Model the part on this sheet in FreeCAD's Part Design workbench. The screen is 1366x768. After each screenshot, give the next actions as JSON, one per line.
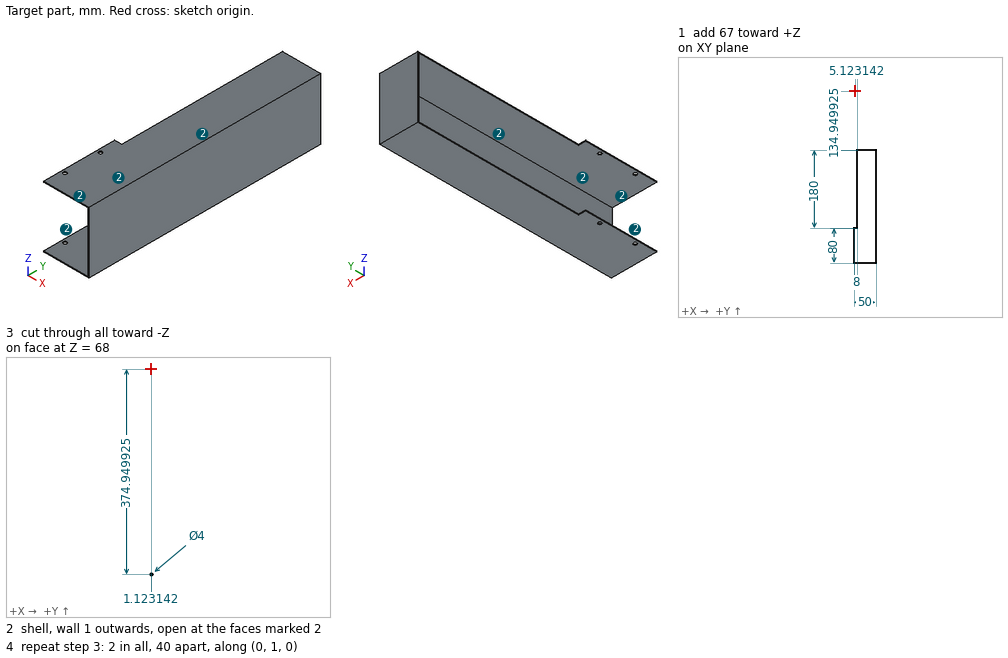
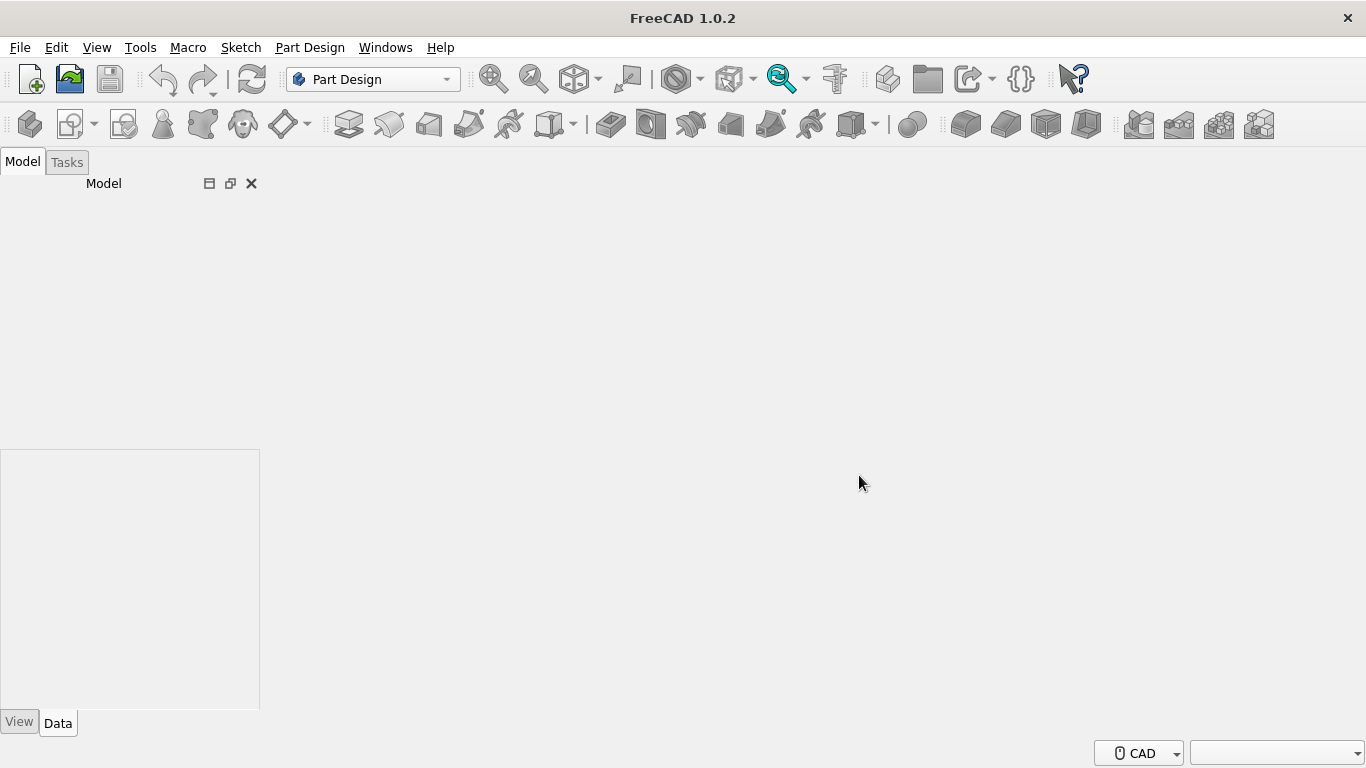
{"action": "left_click", "coordinate": [30, 80]}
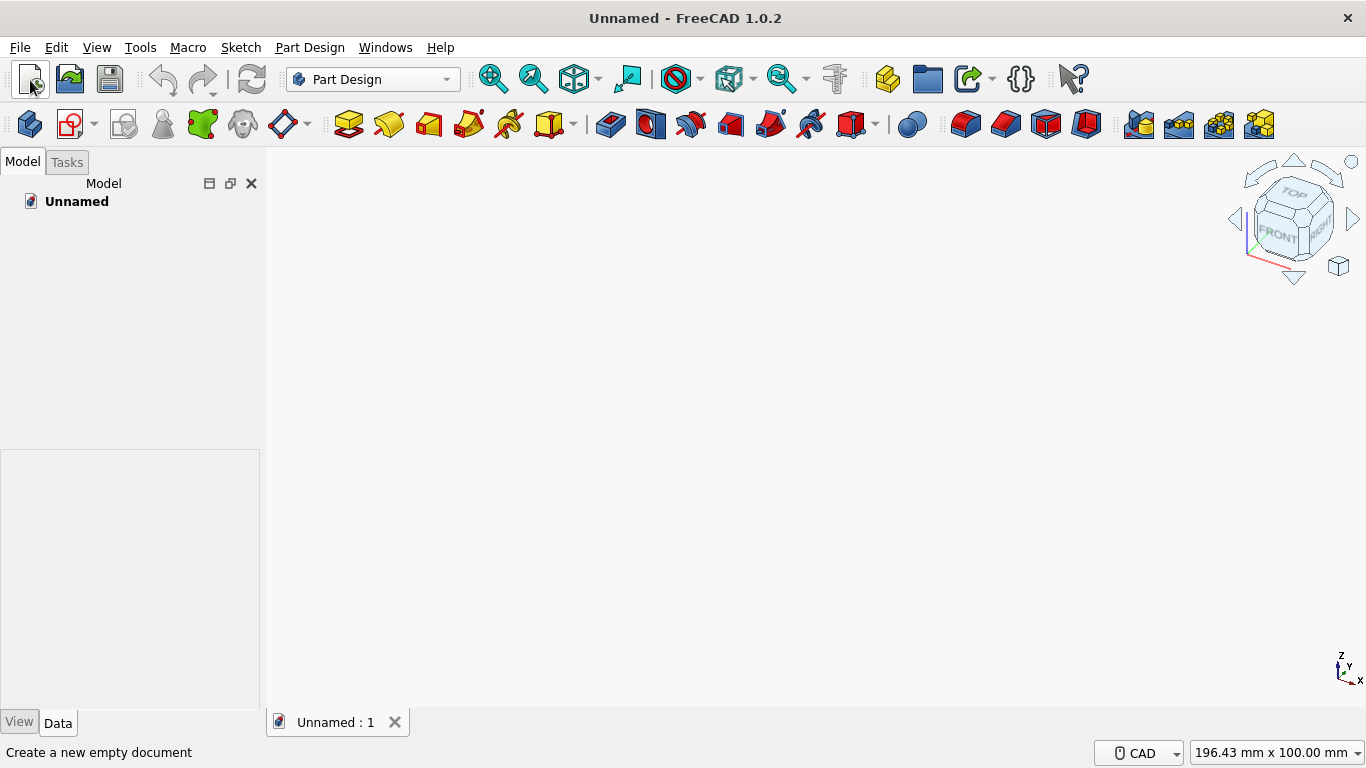
{"action": "left_click", "coordinate": [70, 124]}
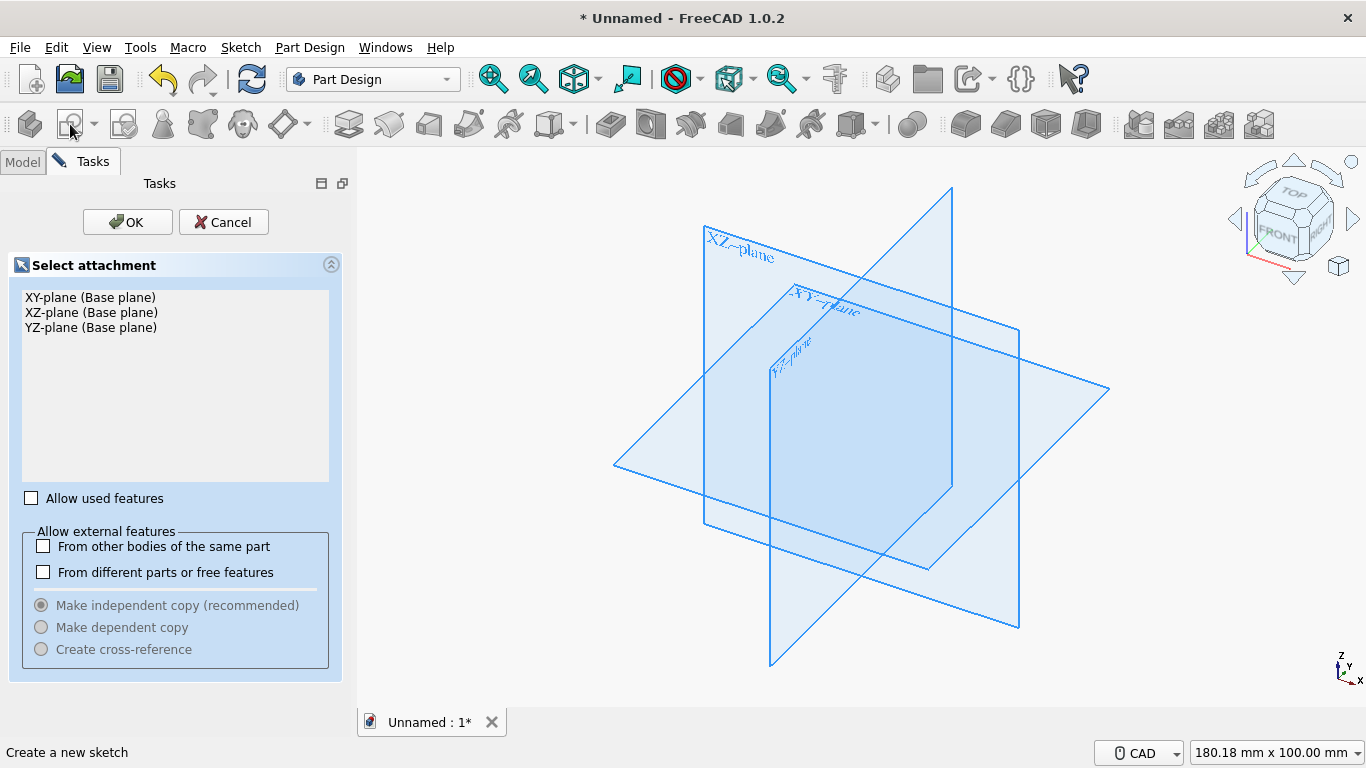
{"action": "left_click", "coordinate": [82, 298]}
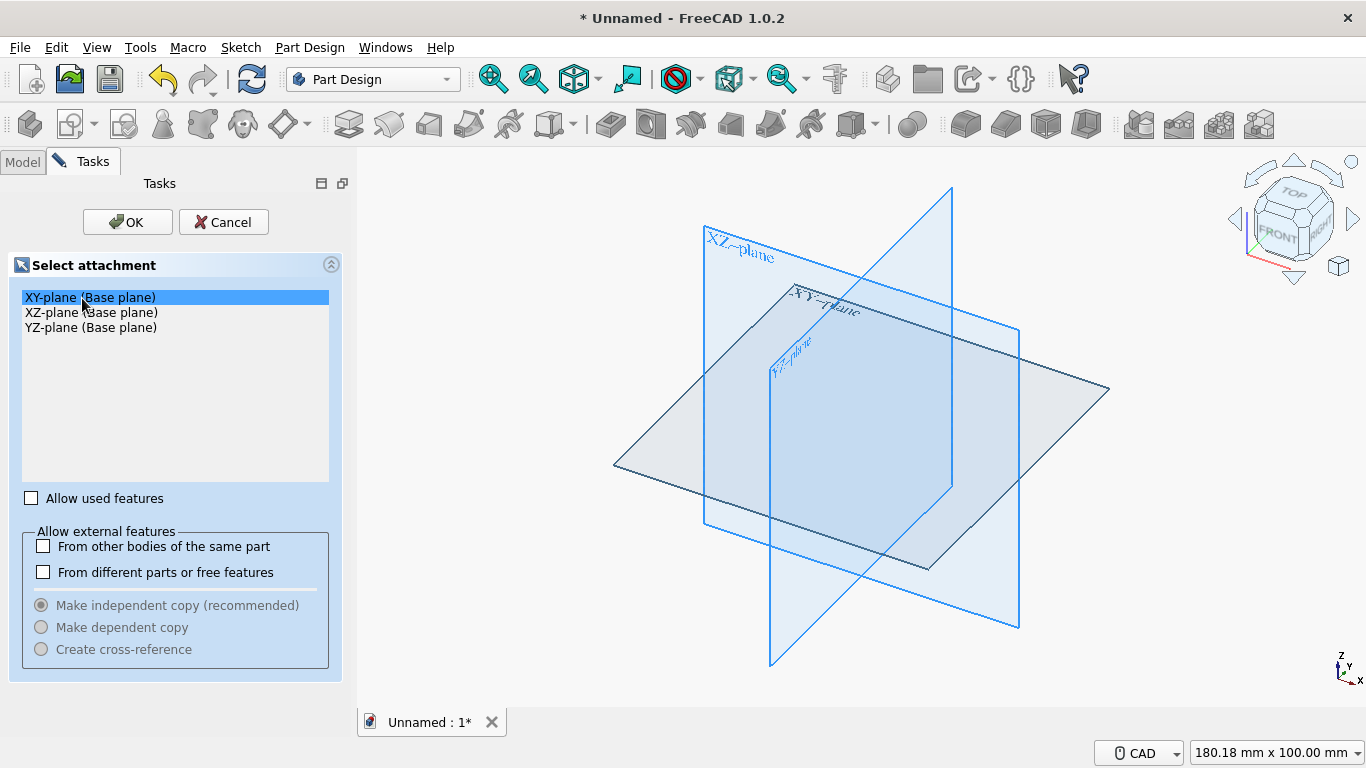
{"action": "left_click", "coordinate": [128, 222]}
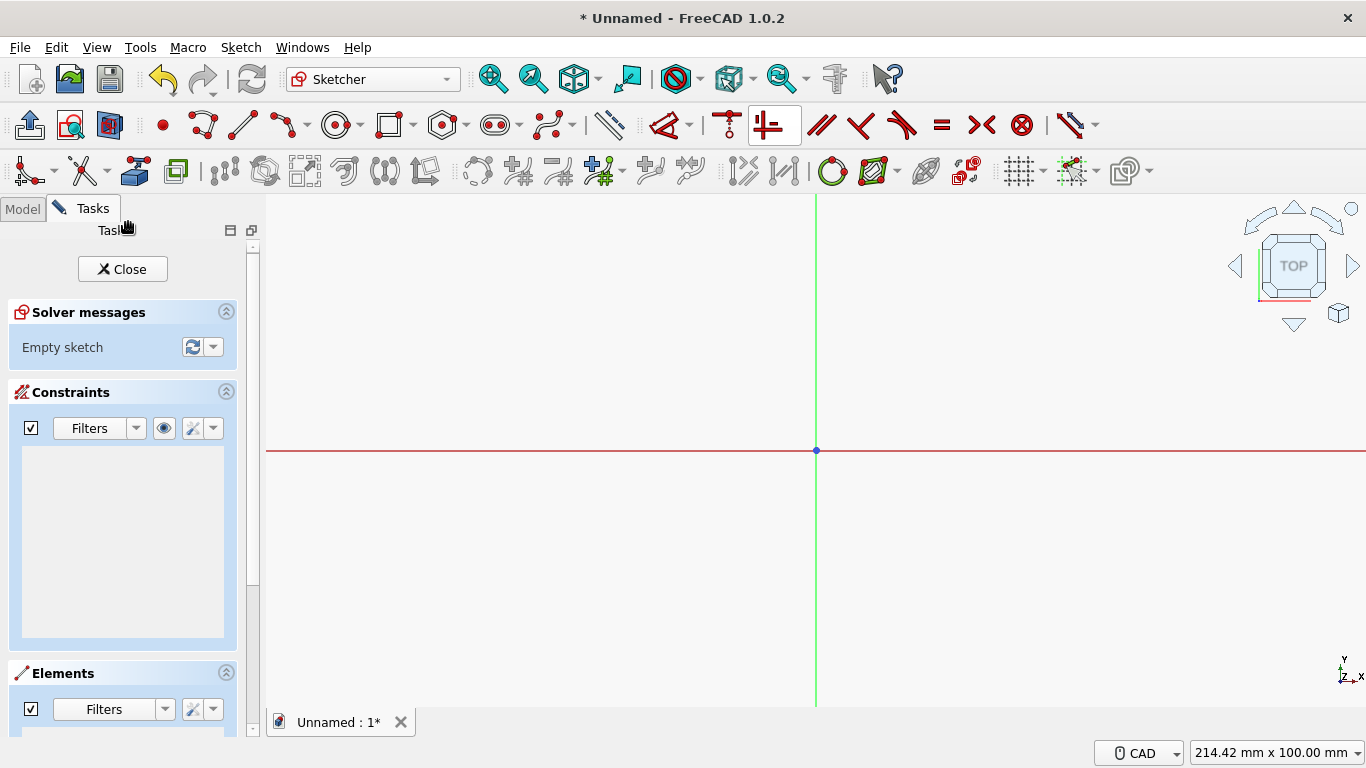
{"action": "scroll", "coordinate": [711, 250], "scroll_direction": "down", "scroll_amount": 9}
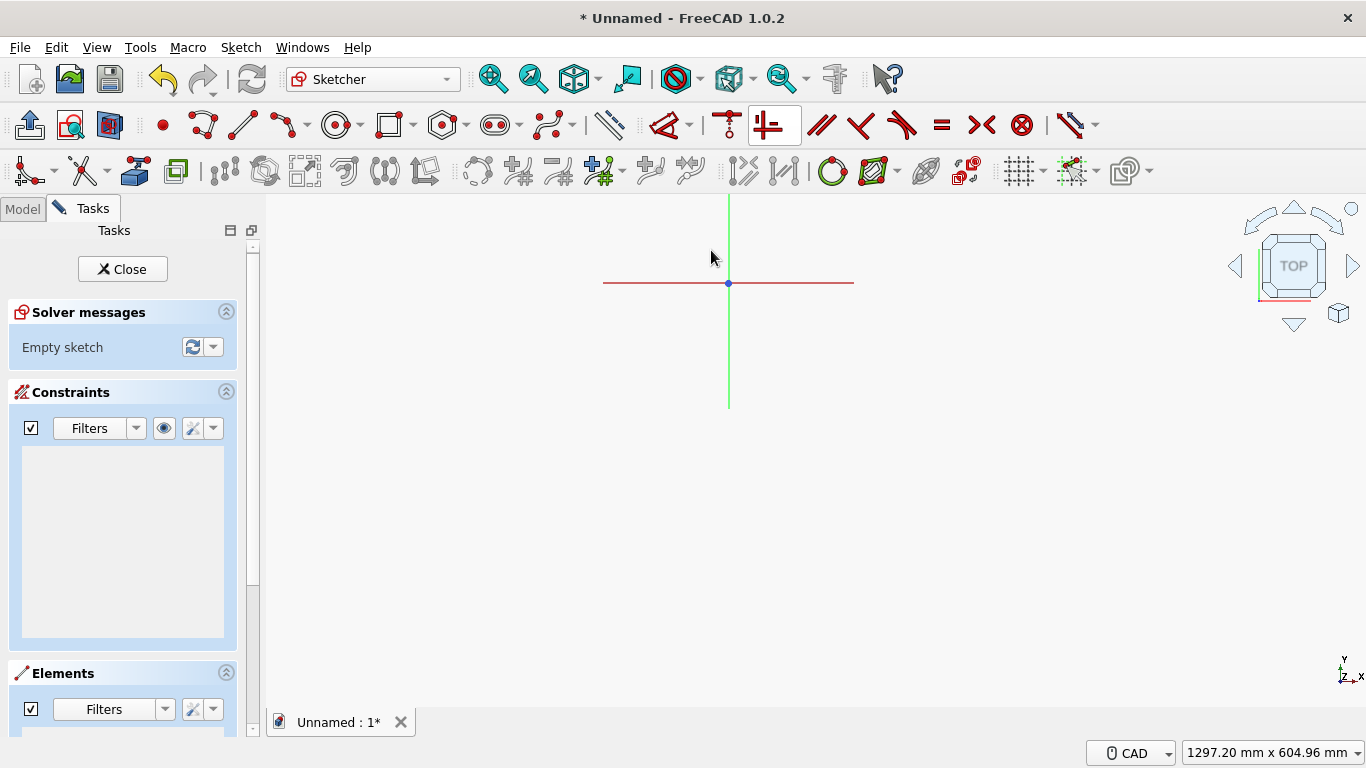
{"action": "left_click", "coordinate": [204, 126]}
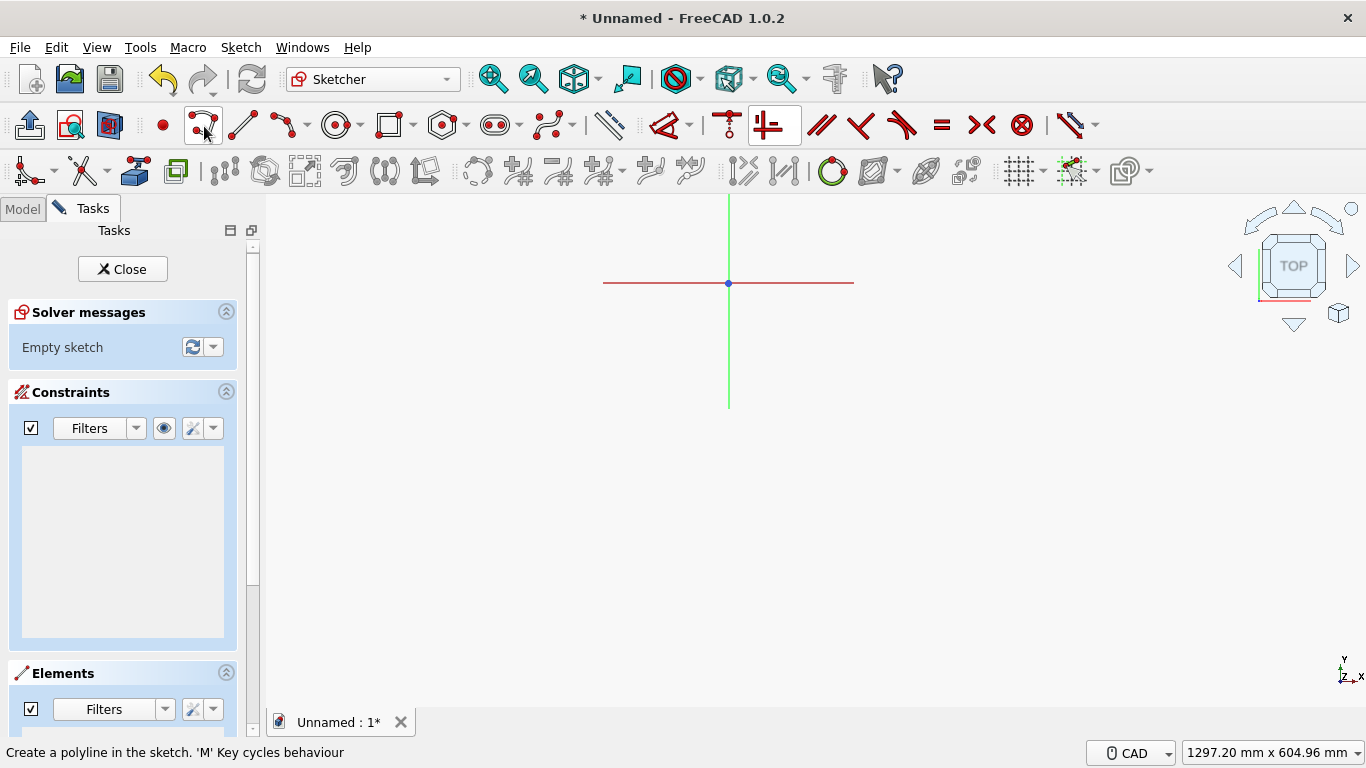
{"action": "scroll", "coordinate": [733, 398], "scroll_direction": "up", "scroll_amount": 7}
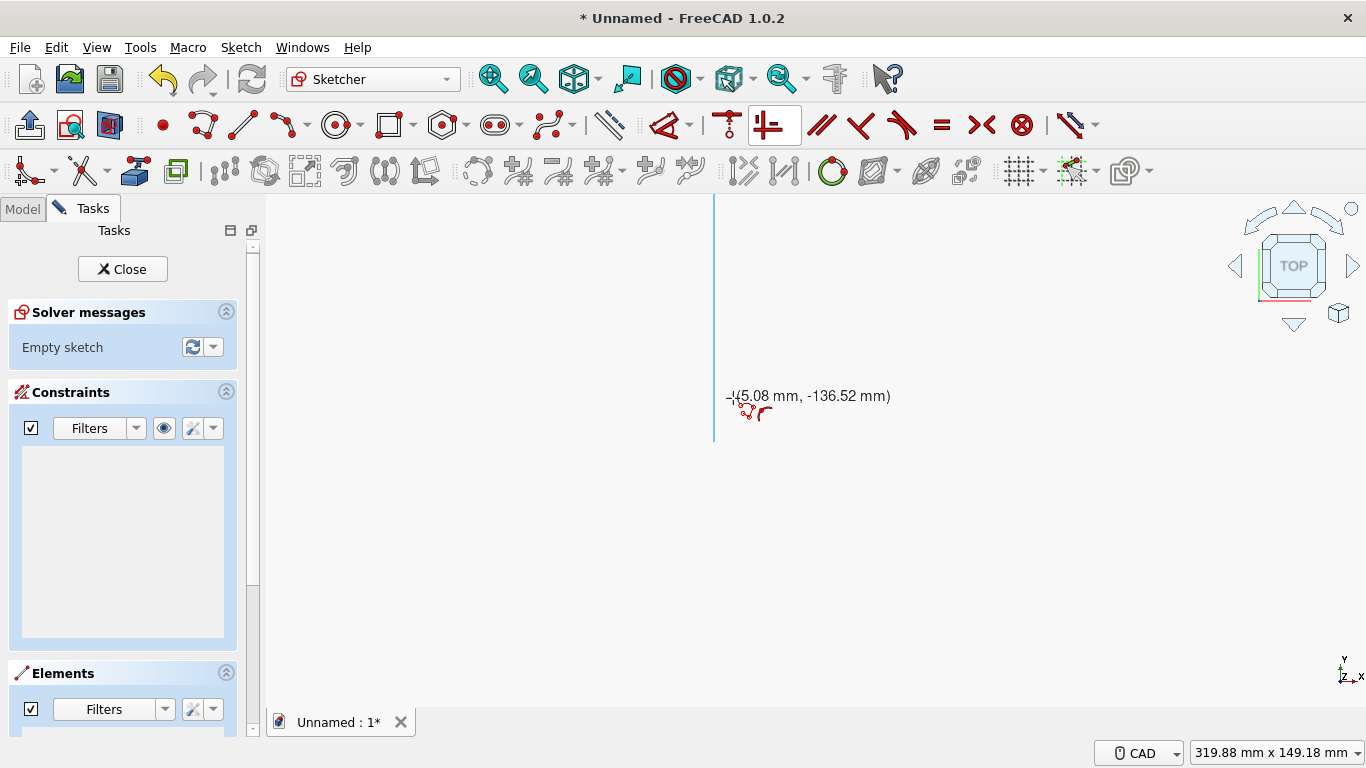
{"action": "left_click", "coordinate": [732, 395]}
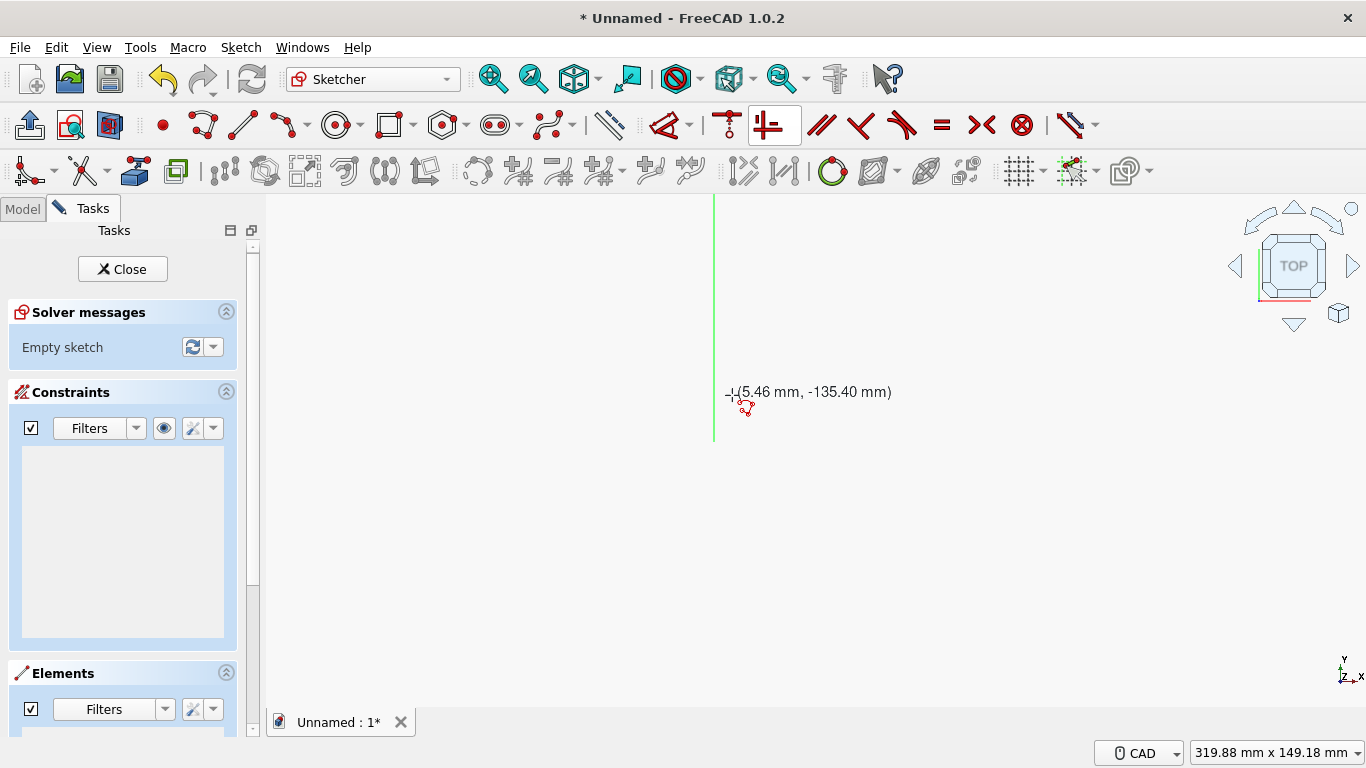
{"action": "scroll", "coordinate": [733, 398], "scroll_direction": "down", "scroll_amount": 7}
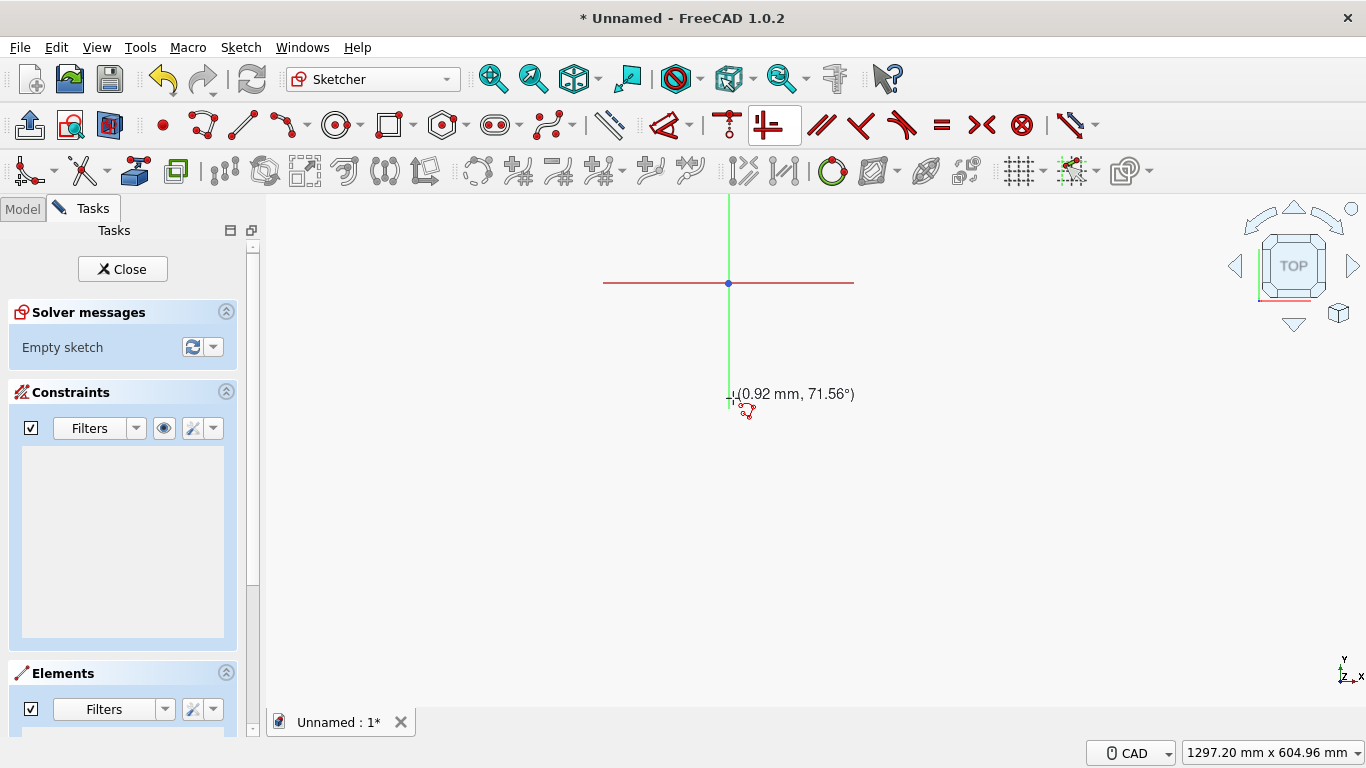
{"action": "scroll", "coordinate": [733, 550], "scroll_direction": "up", "scroll_amount": 7}